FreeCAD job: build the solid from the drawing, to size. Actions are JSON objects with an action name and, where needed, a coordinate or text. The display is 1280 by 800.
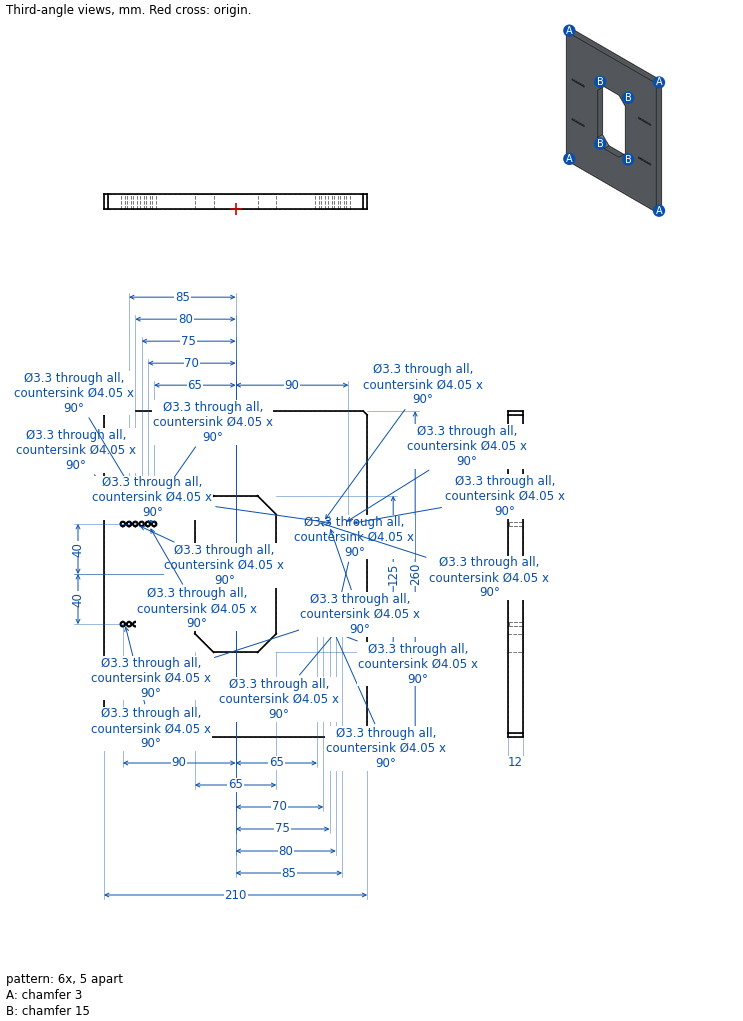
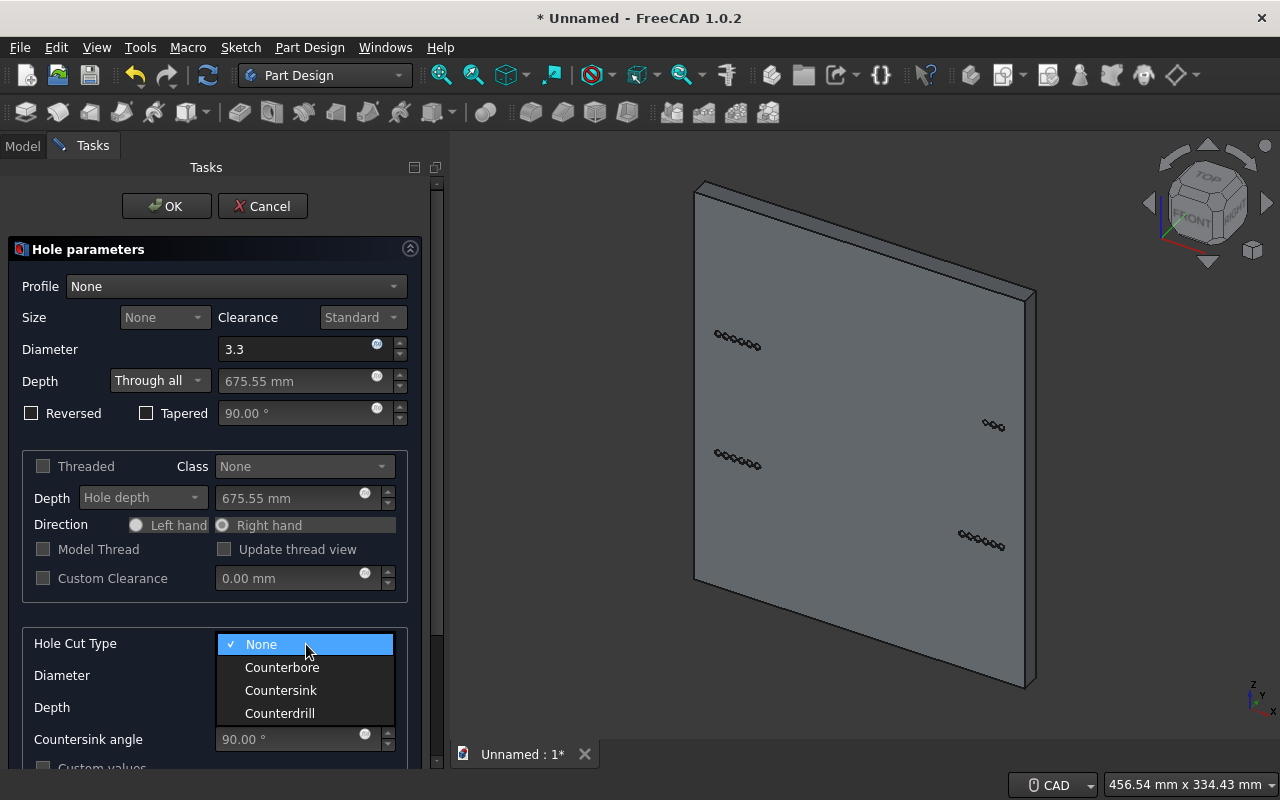
{"action": "left_click", "coordinate": [304, 690]}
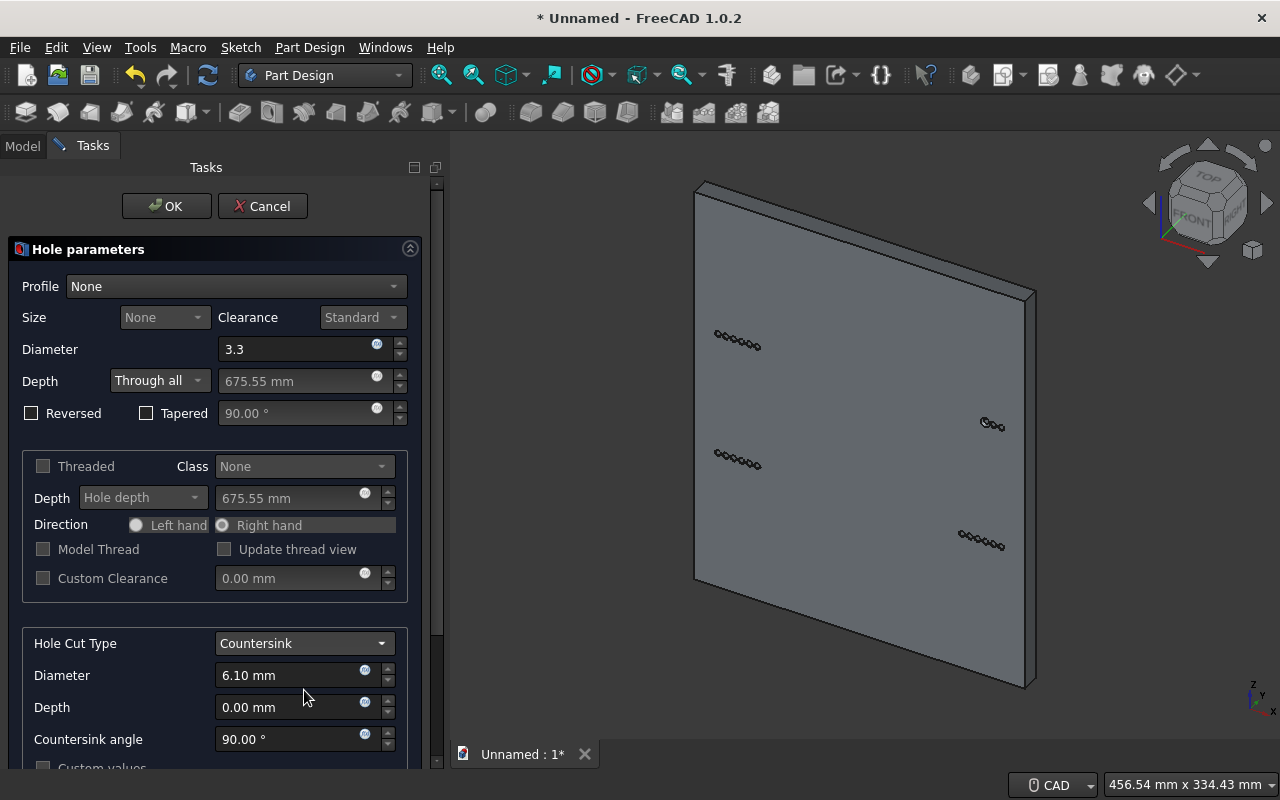
{"action": "triple_click", "coordinate": [298, 675]}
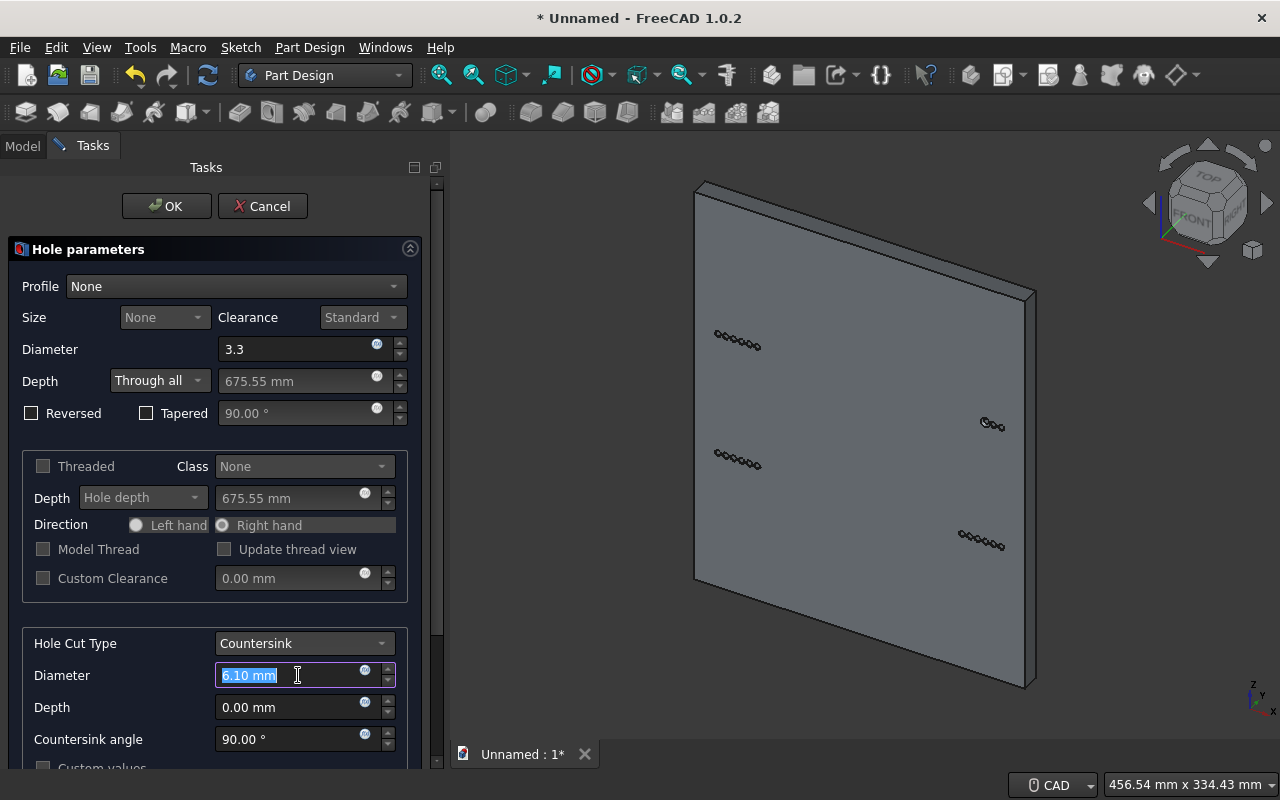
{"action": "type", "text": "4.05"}
{"action": "key", "text": "Tab"}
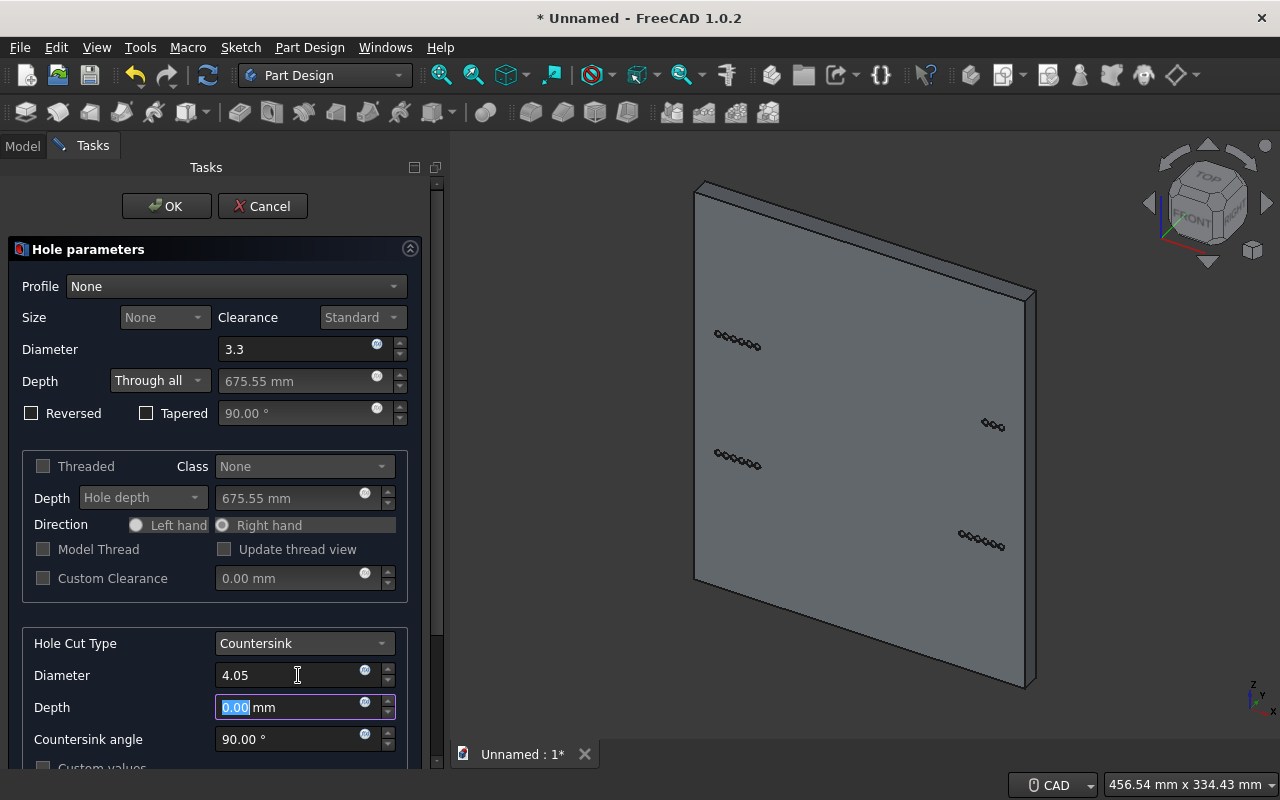
{"action": "left_click", "coordinate": [167, 206]}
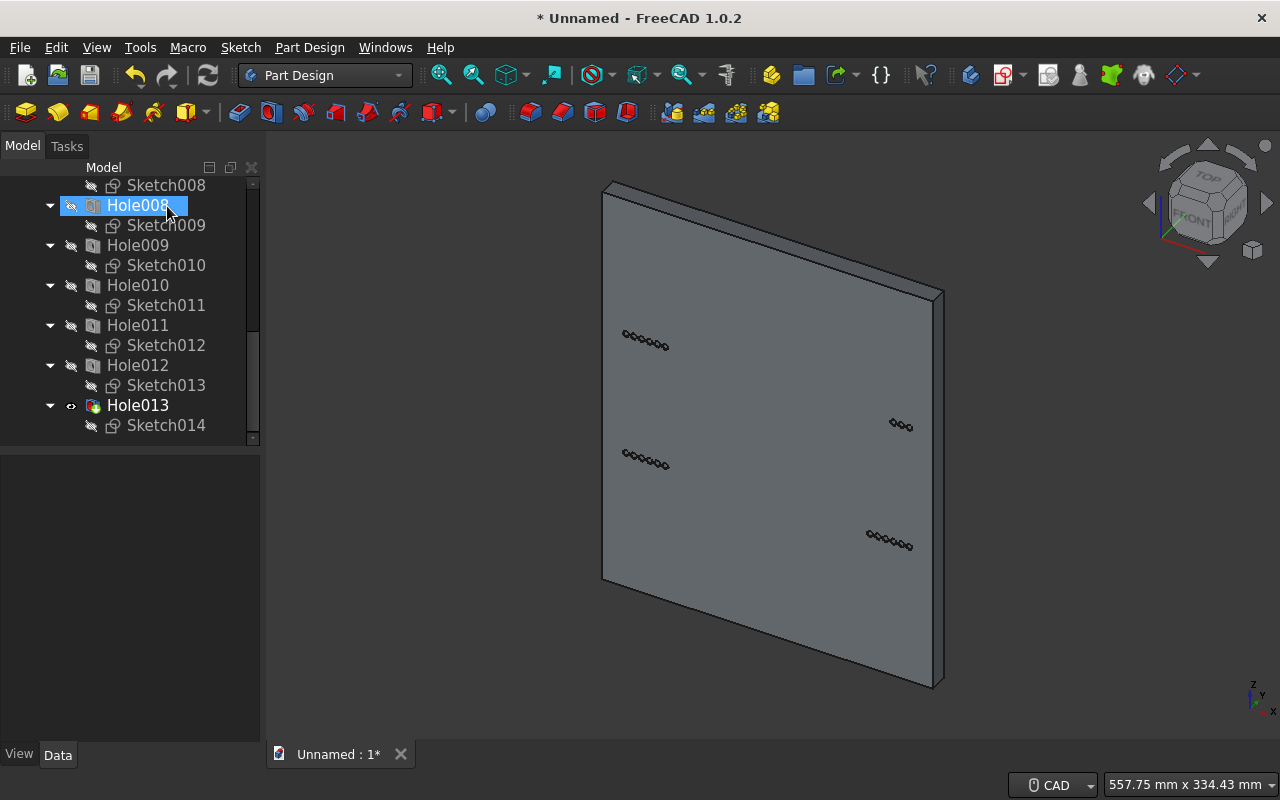
{"action": "left_click", "coordinate": [768, 439]}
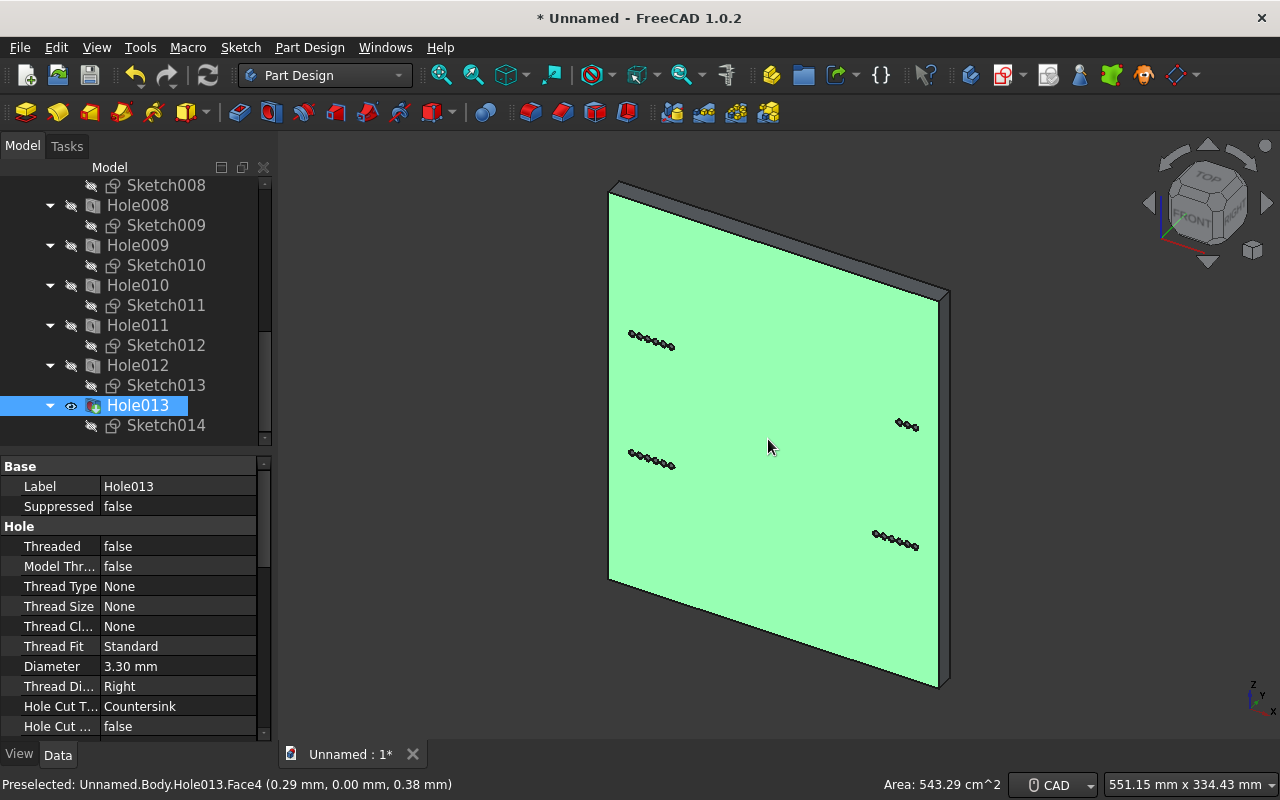
{"action": "left_click", "coordinate": [1004, 76]}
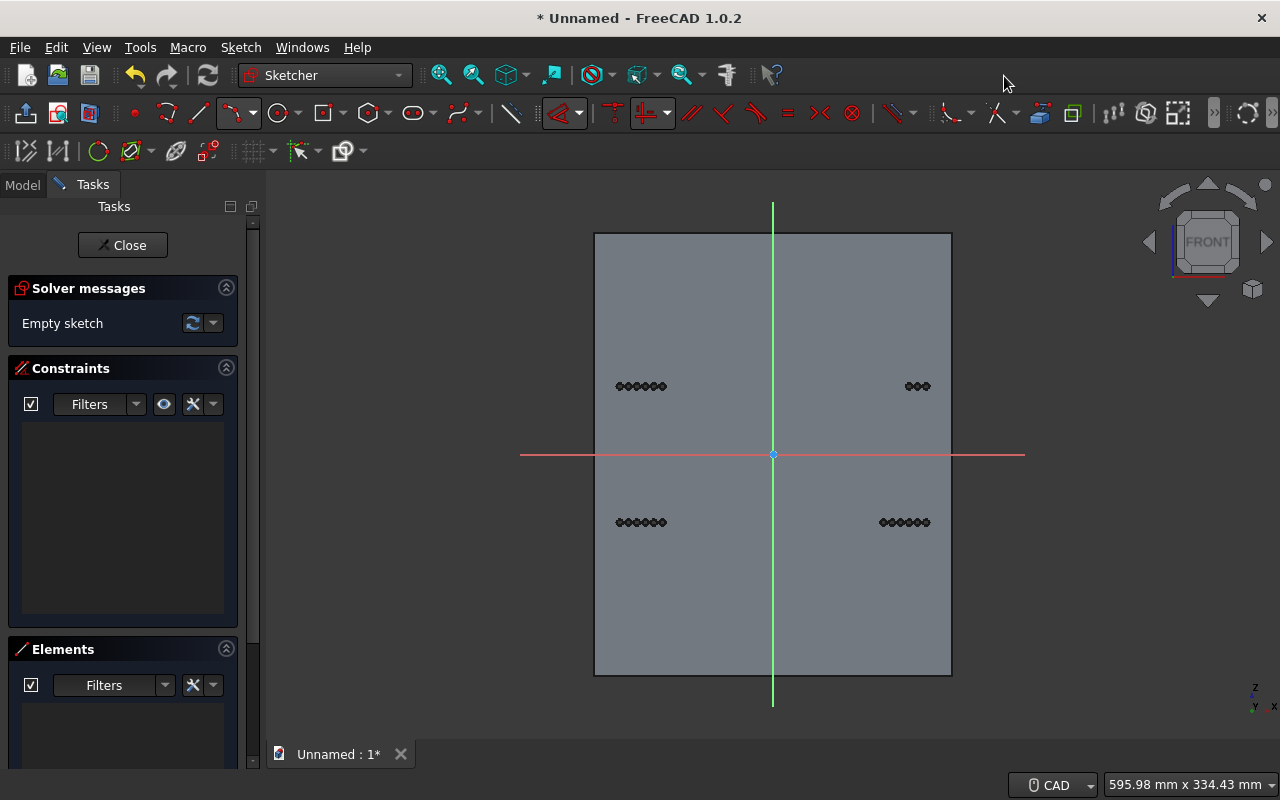
{"action": "scroll", "coordinate": [911, 383], "scroll_direction": "up", "scroll_amount": 15}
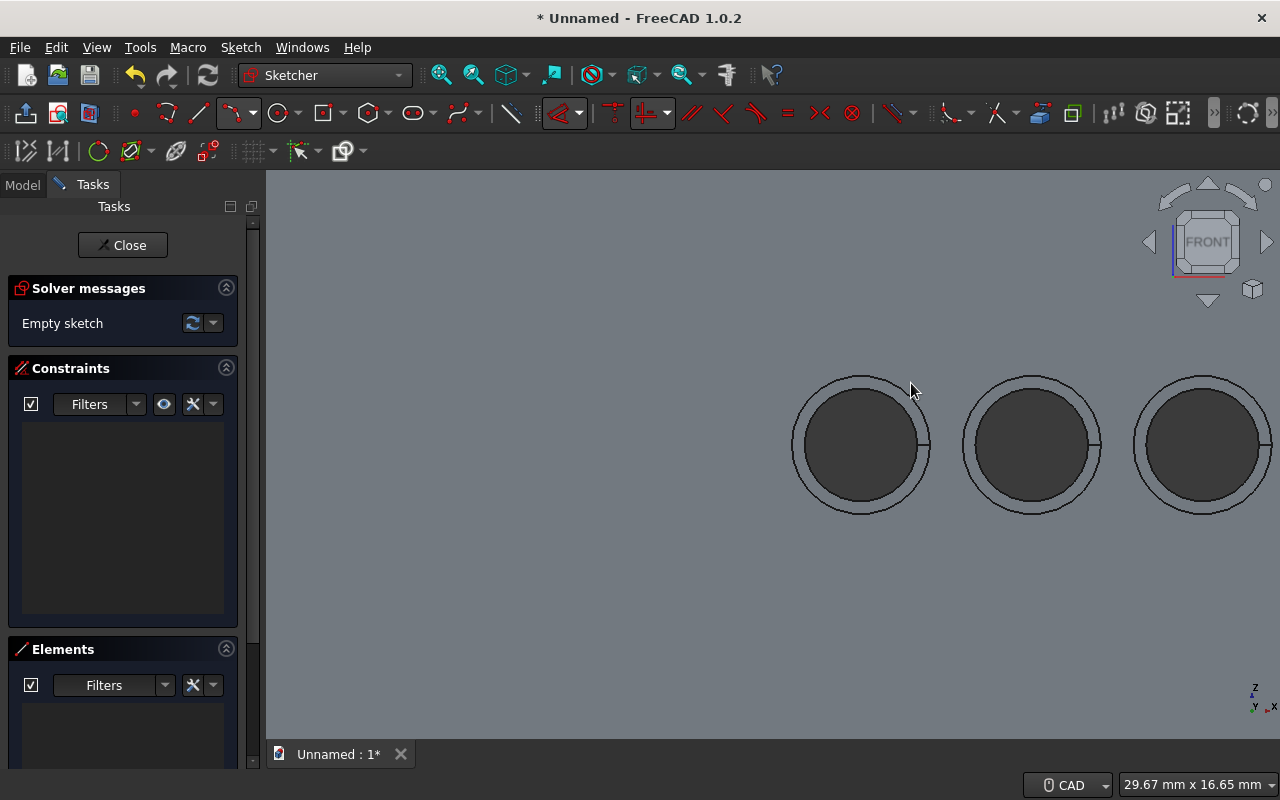
{"action": "scroll", "coordinate": [684, 441], "scroll_direction": "up", "scroll_amount": 6}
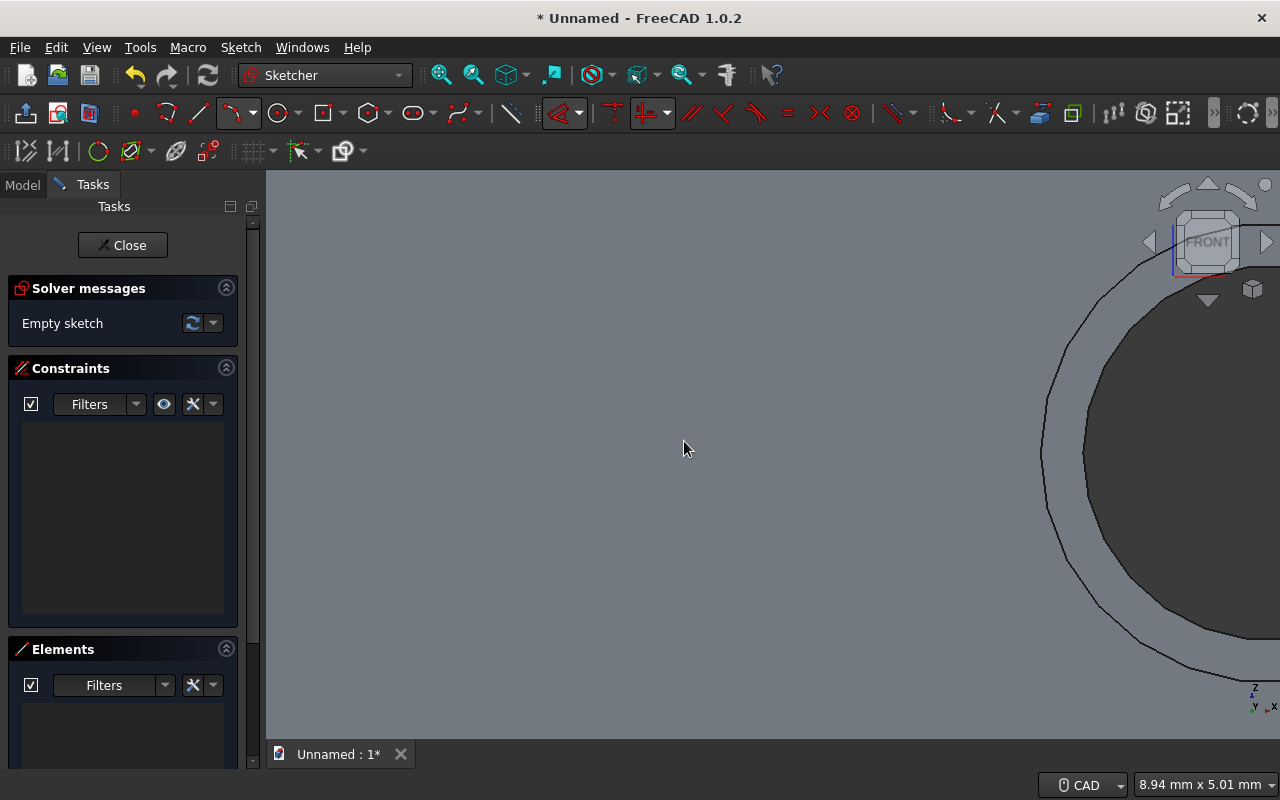
{"action": "left_click", "coordinate": [278, 114]}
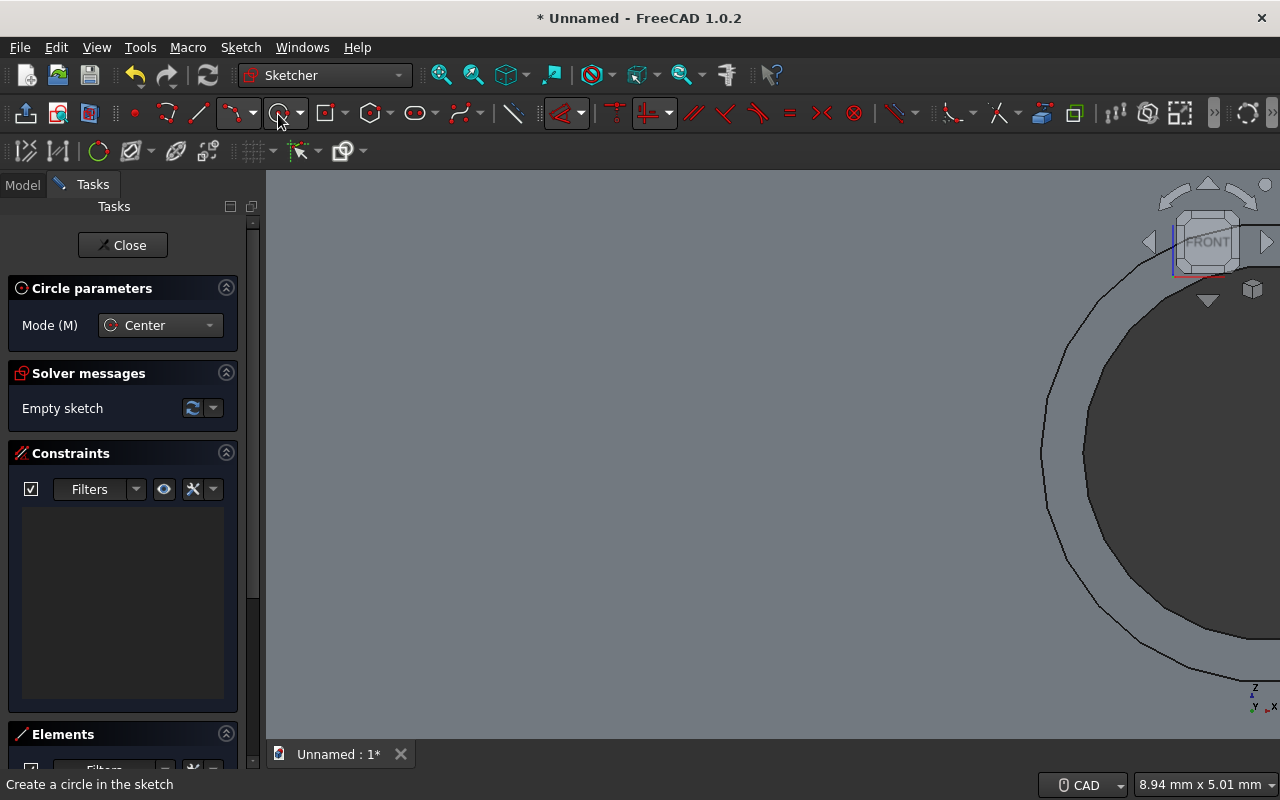
{"action": "left_click", "coordinate": [703, 453]}
{"action": "mouse_move", "coordinate": [836, 321]}